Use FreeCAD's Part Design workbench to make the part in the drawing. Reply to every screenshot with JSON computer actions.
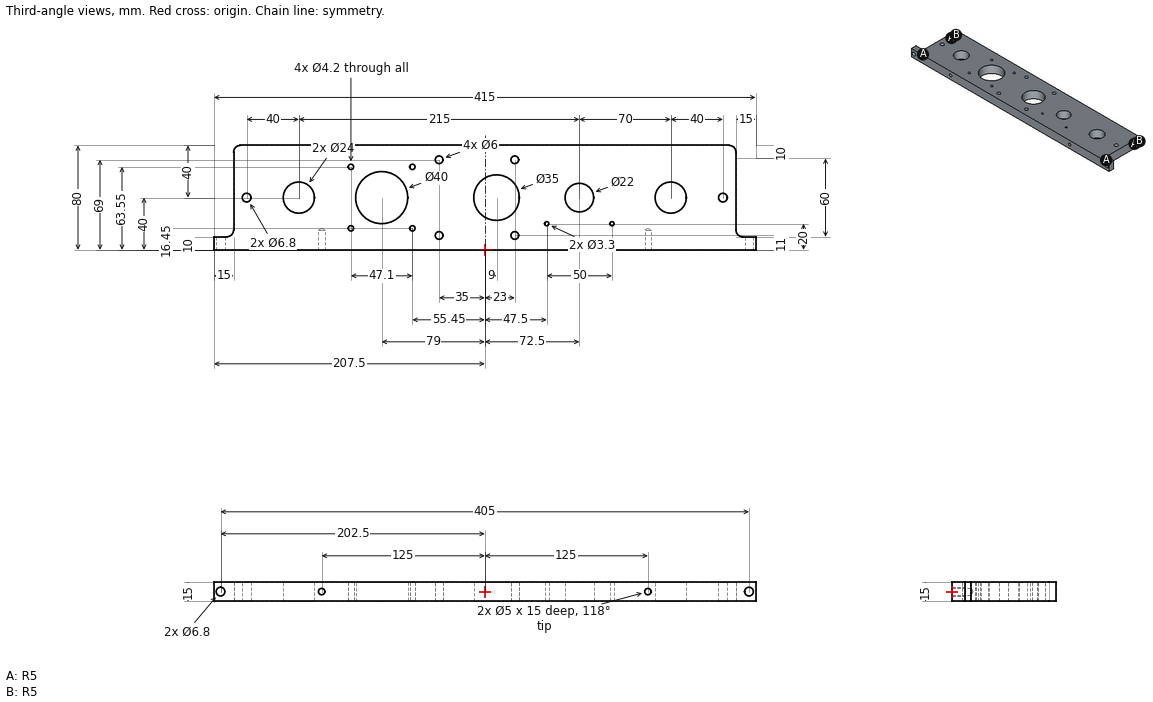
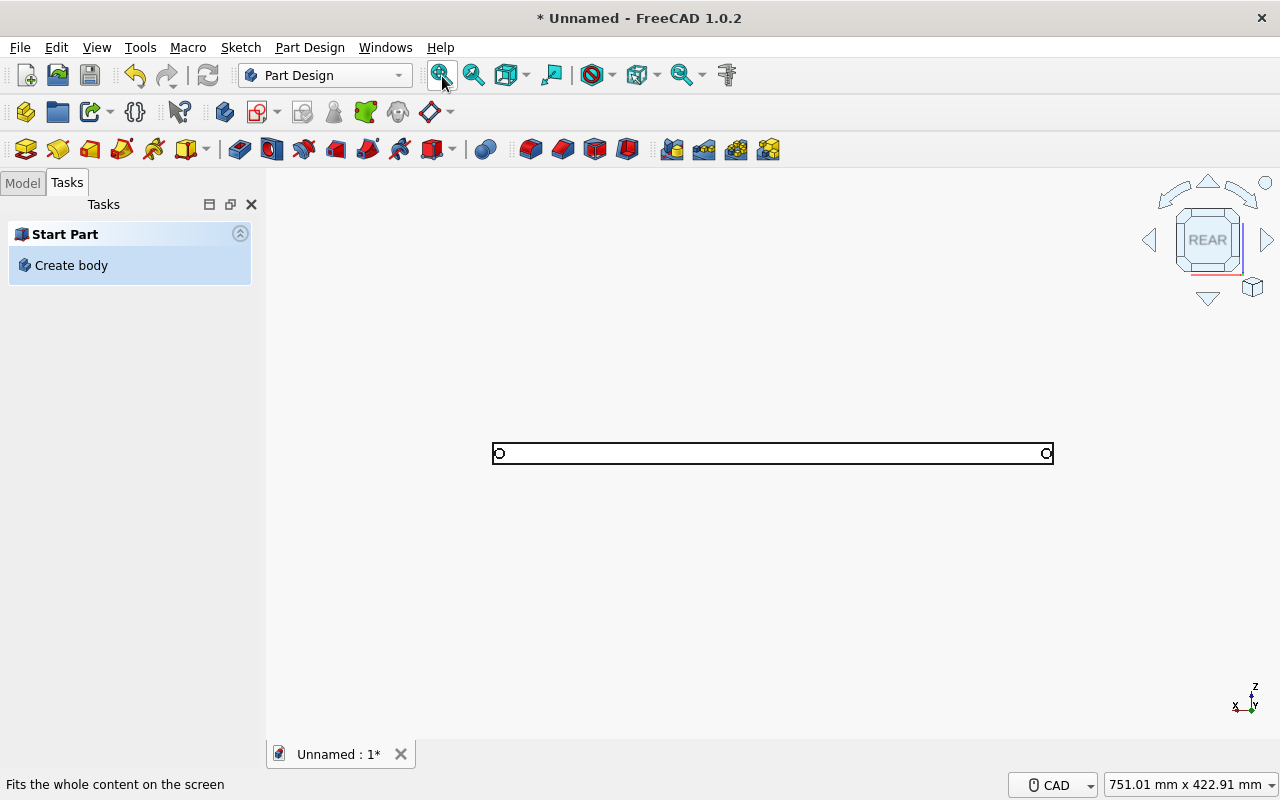
{"action": "key", "text": "0"}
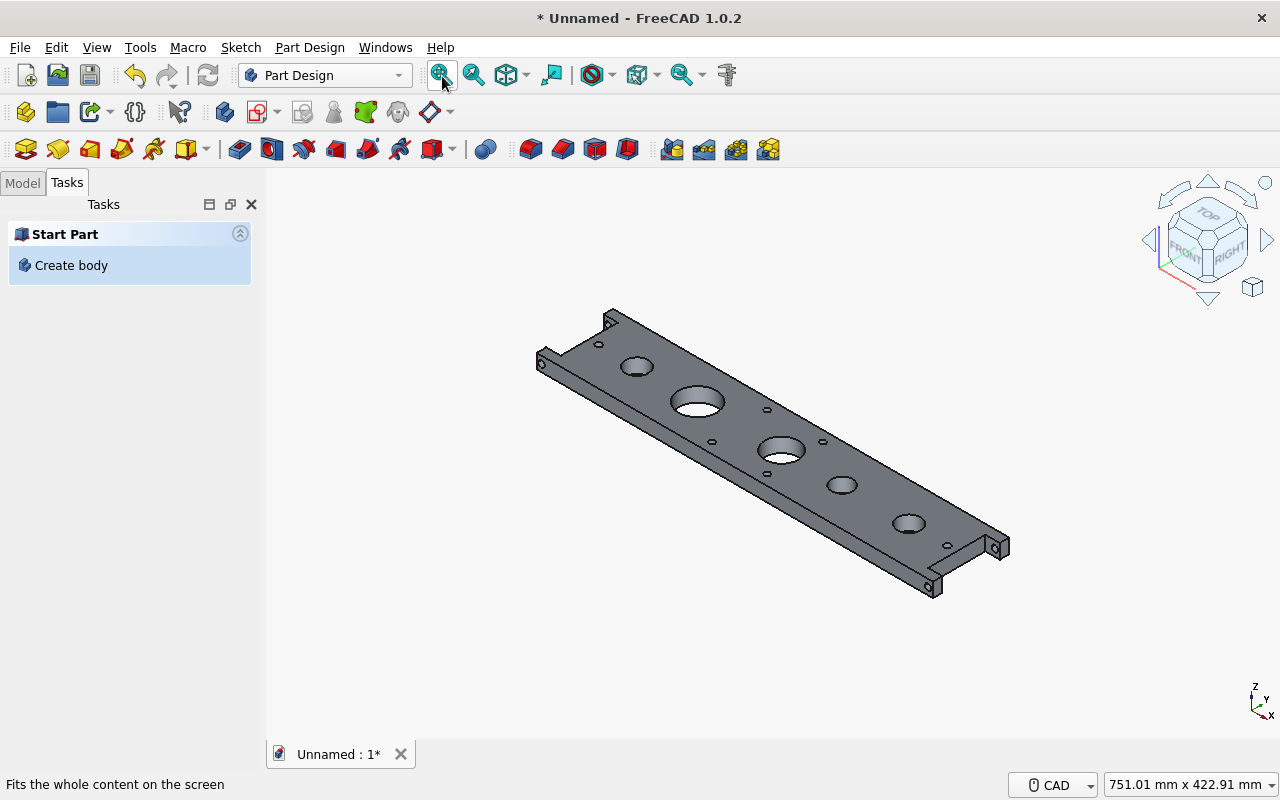
{"action": "scroll", "coordinate": [561, 363], "scroll_direction": "up", "scroll_amount": 4}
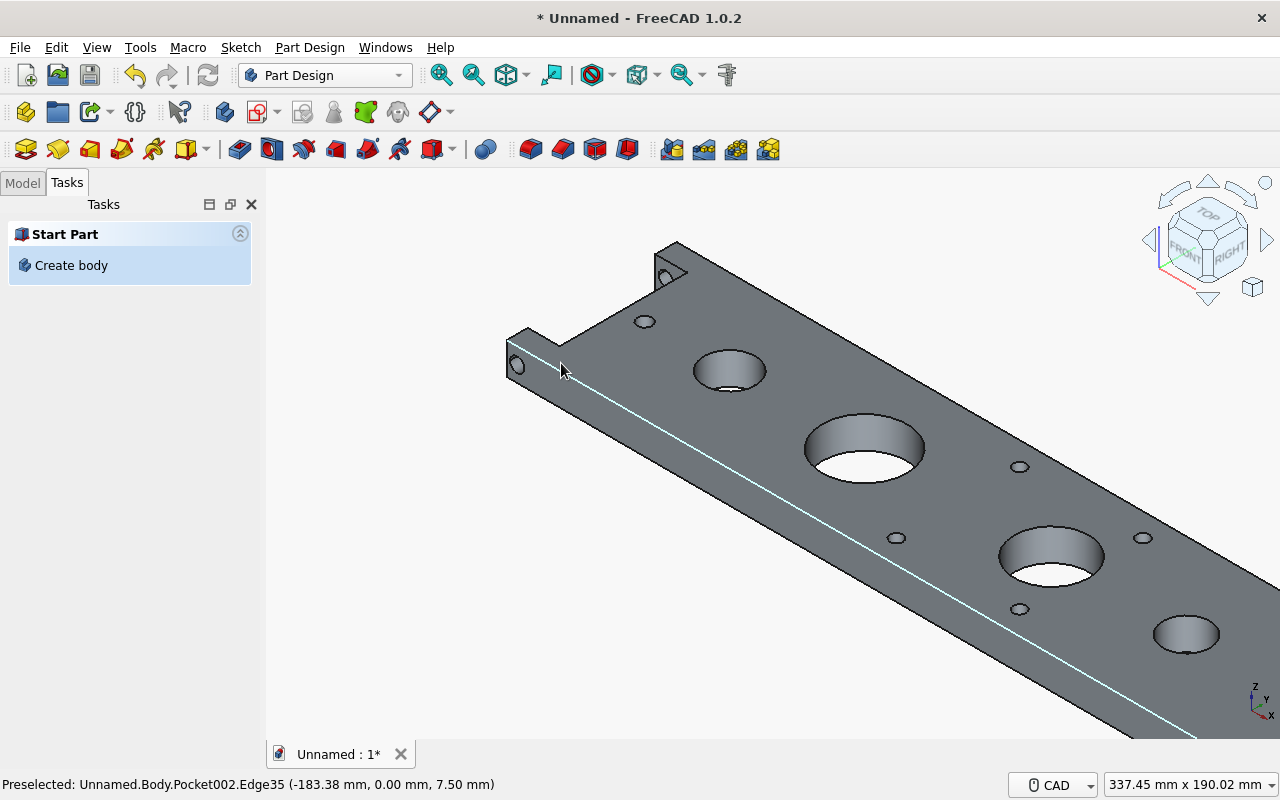
{"action": "left_click", "coordinate": [442, 76]}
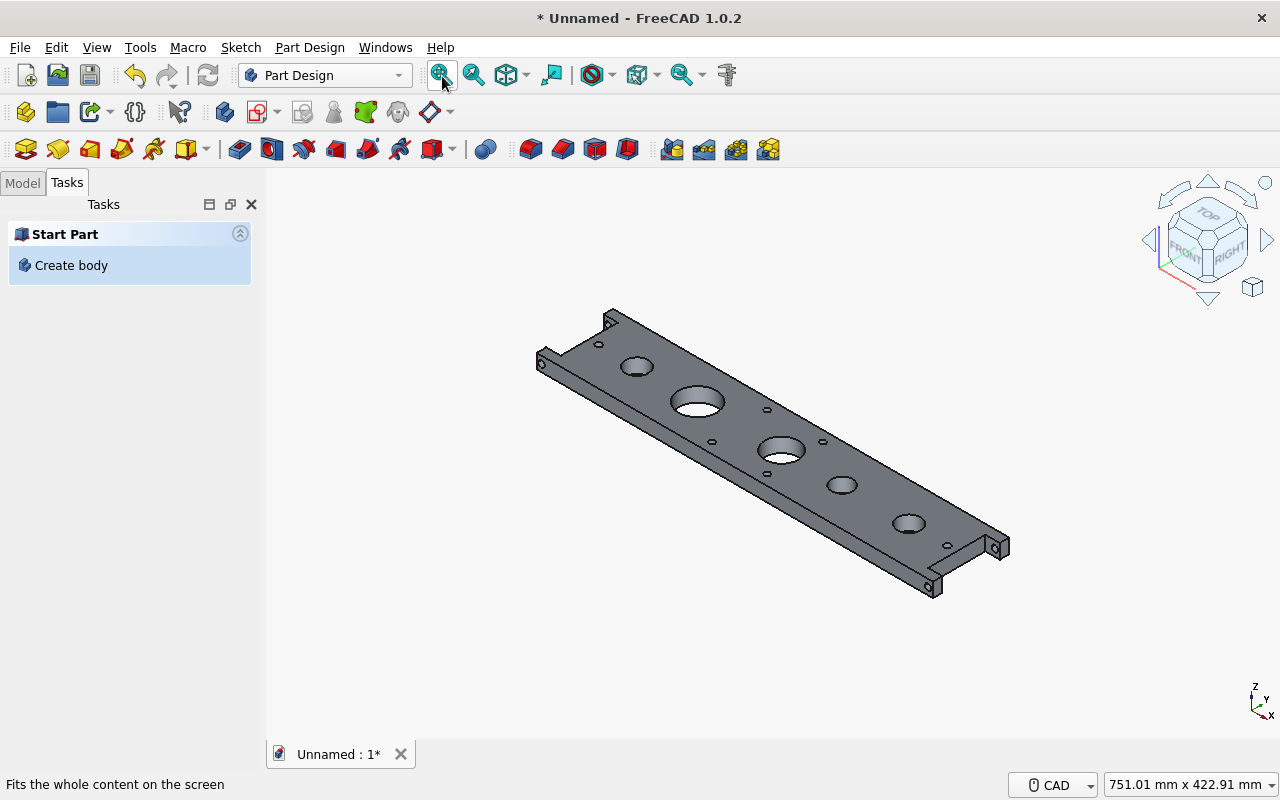
{"action": "key", "text": "2"}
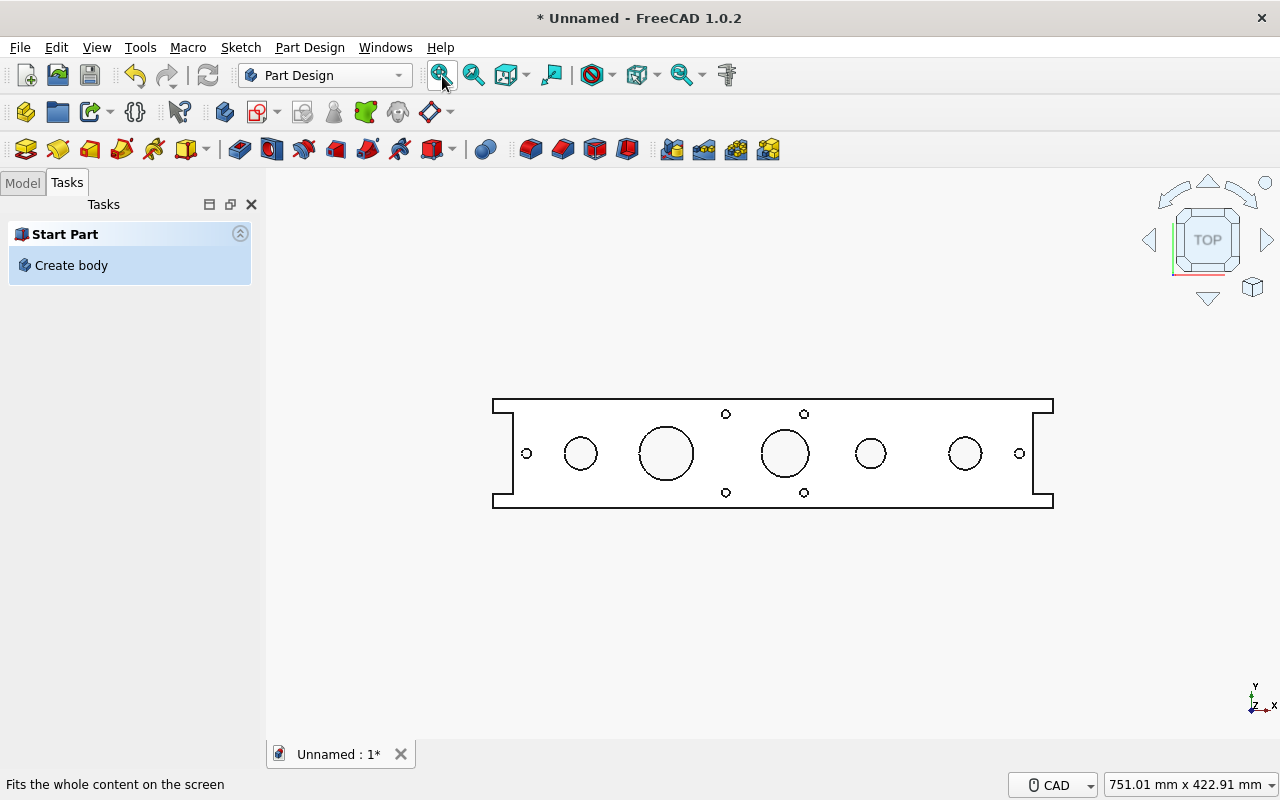
{"action": "scroll", "coordinate": [513, 493], "scroll_direction": "up", "scroll_amount": 4}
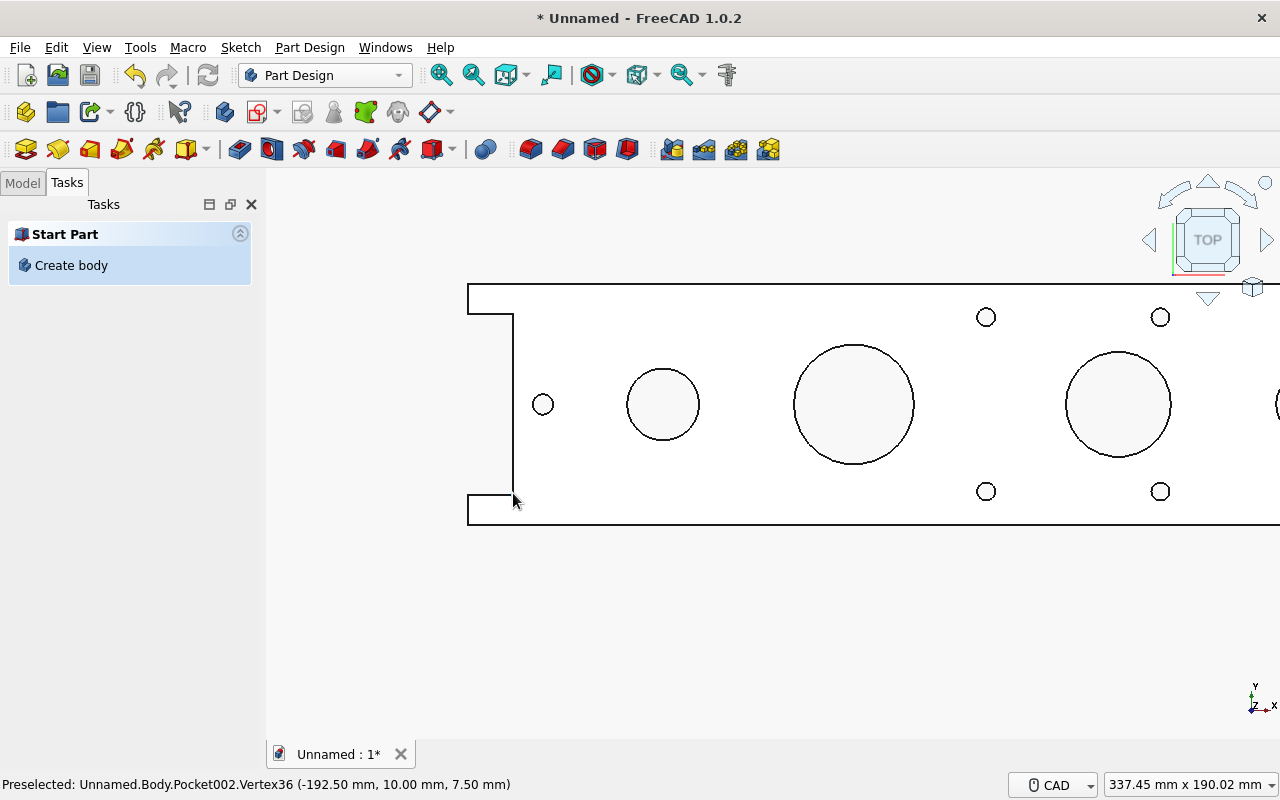
{"action": "left_click", "coordinate": [442, 76]}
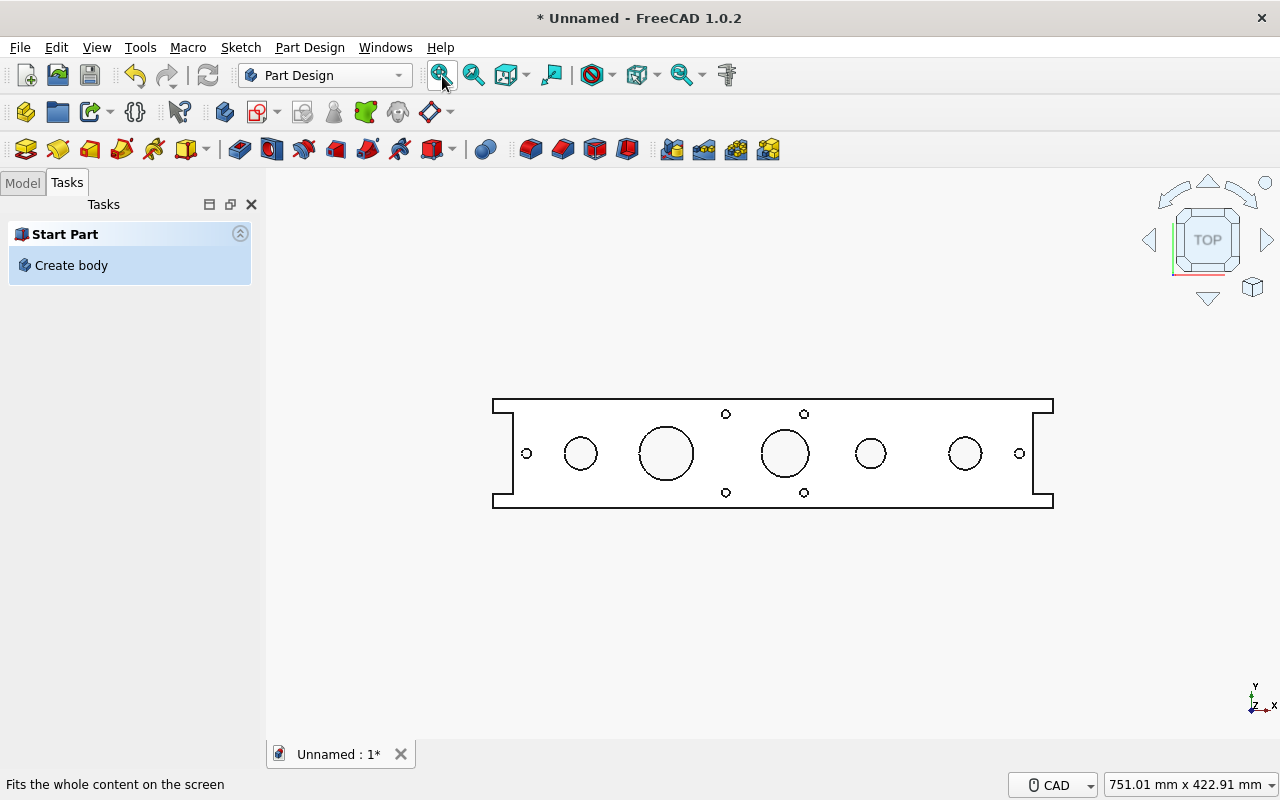
{"action": "key", "text": "1"}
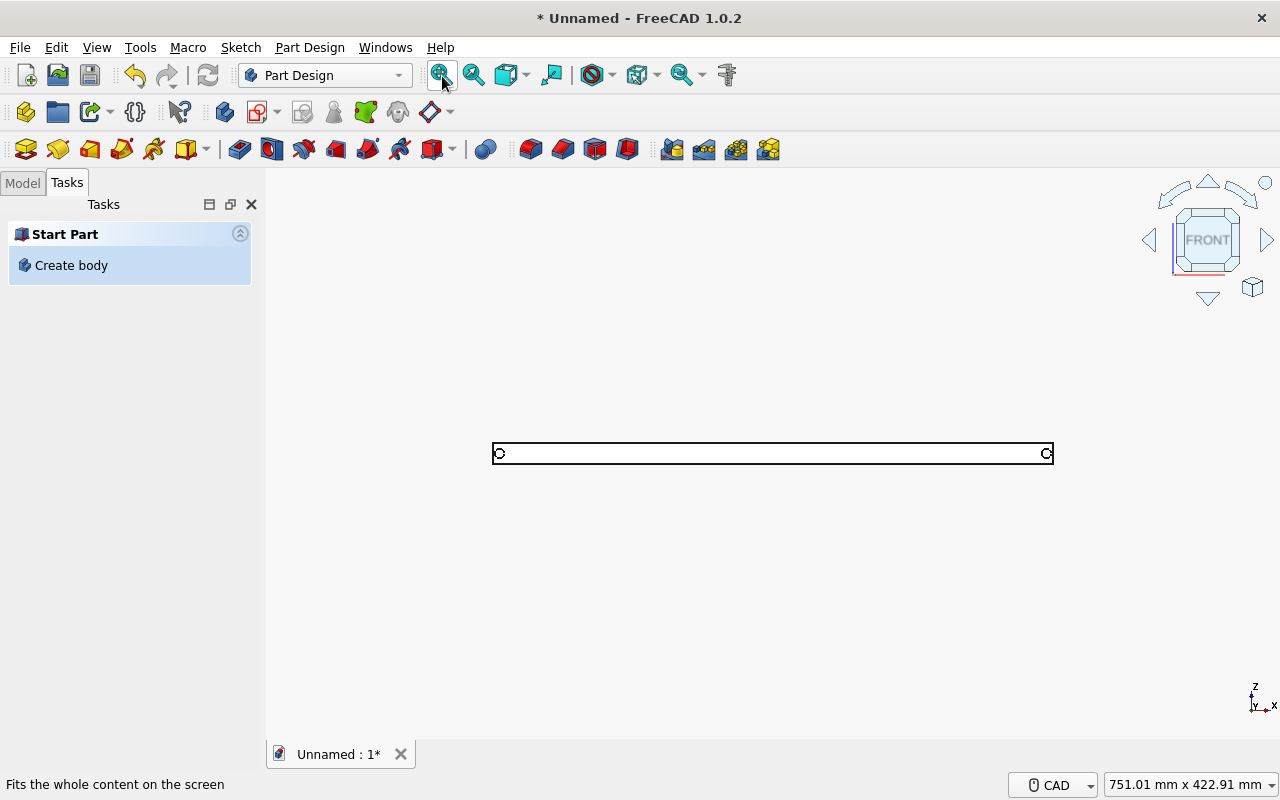
{"action": "scroll", "coordinate": [513, 452], "scroll_direction": "up", "scroll_amount": 4}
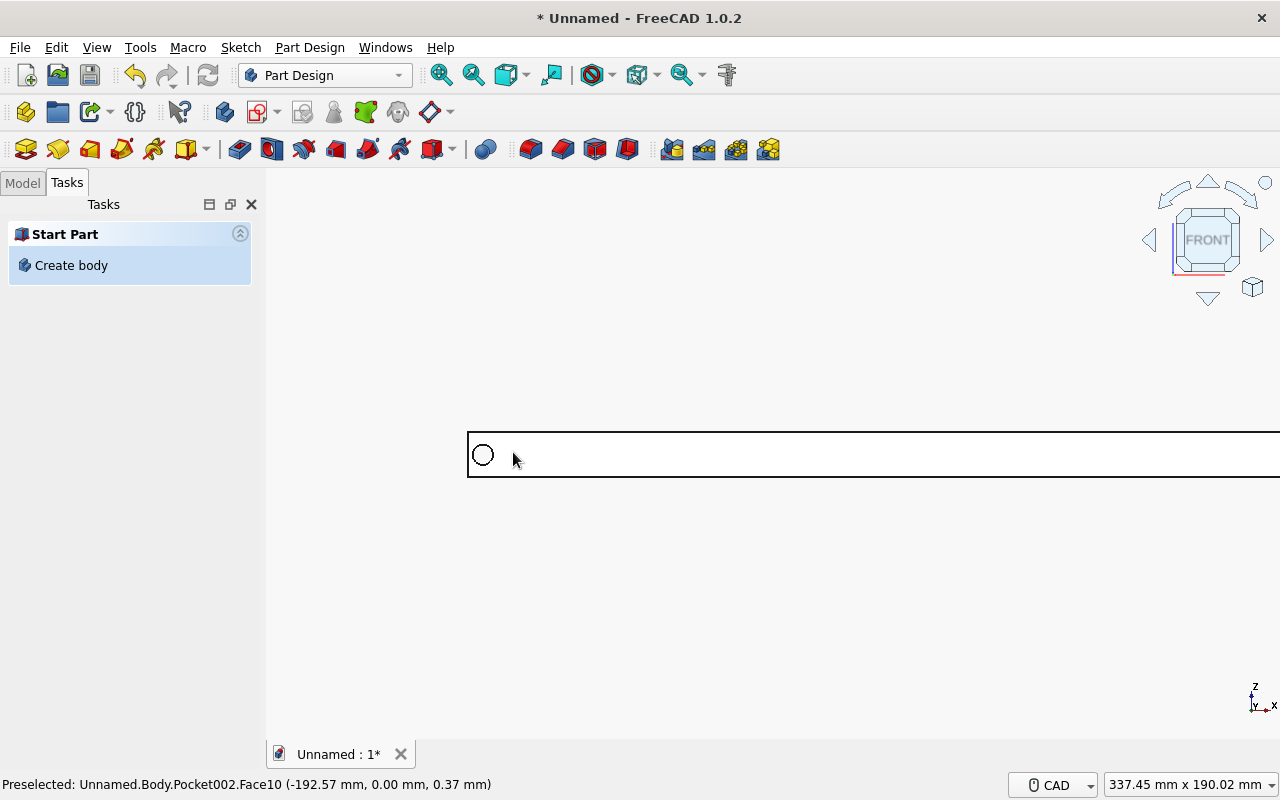
{"action": "left_click", "coordinate": [442, 76]}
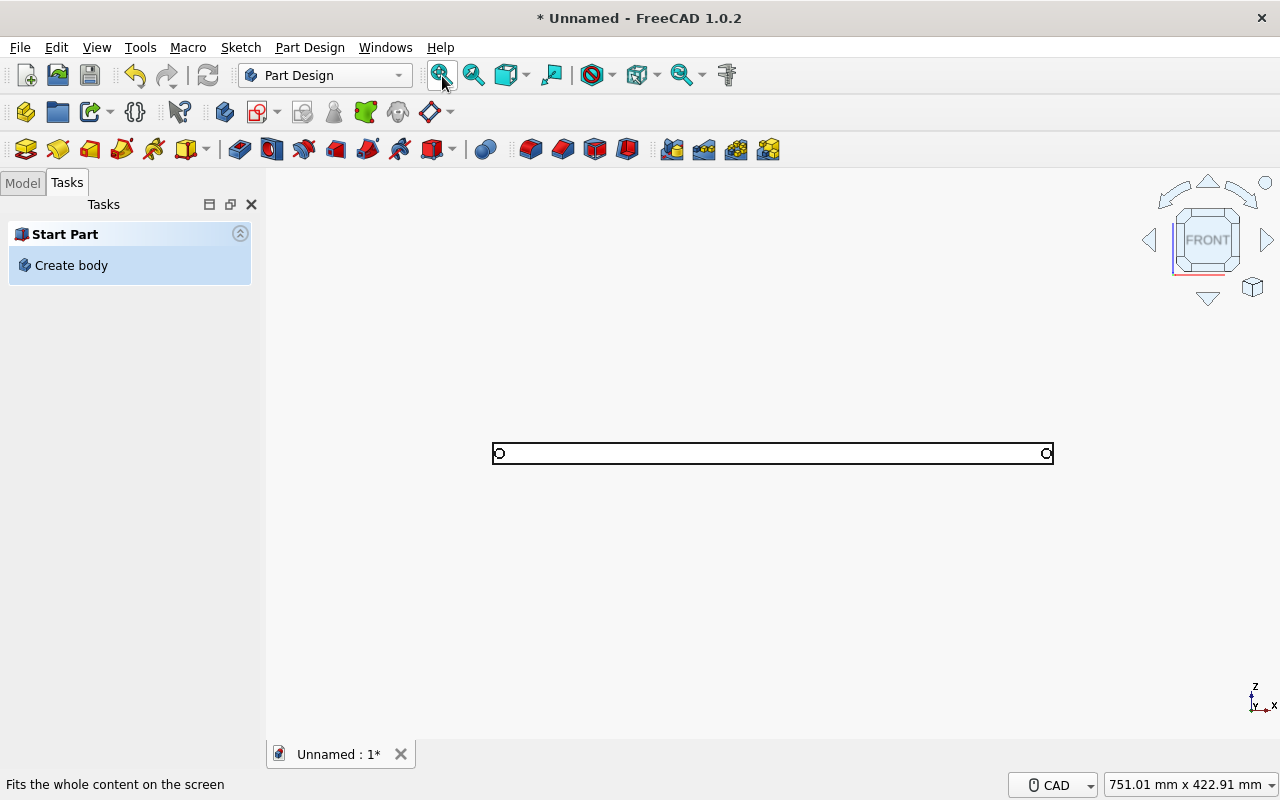
{"action": "key", "text": "3"}